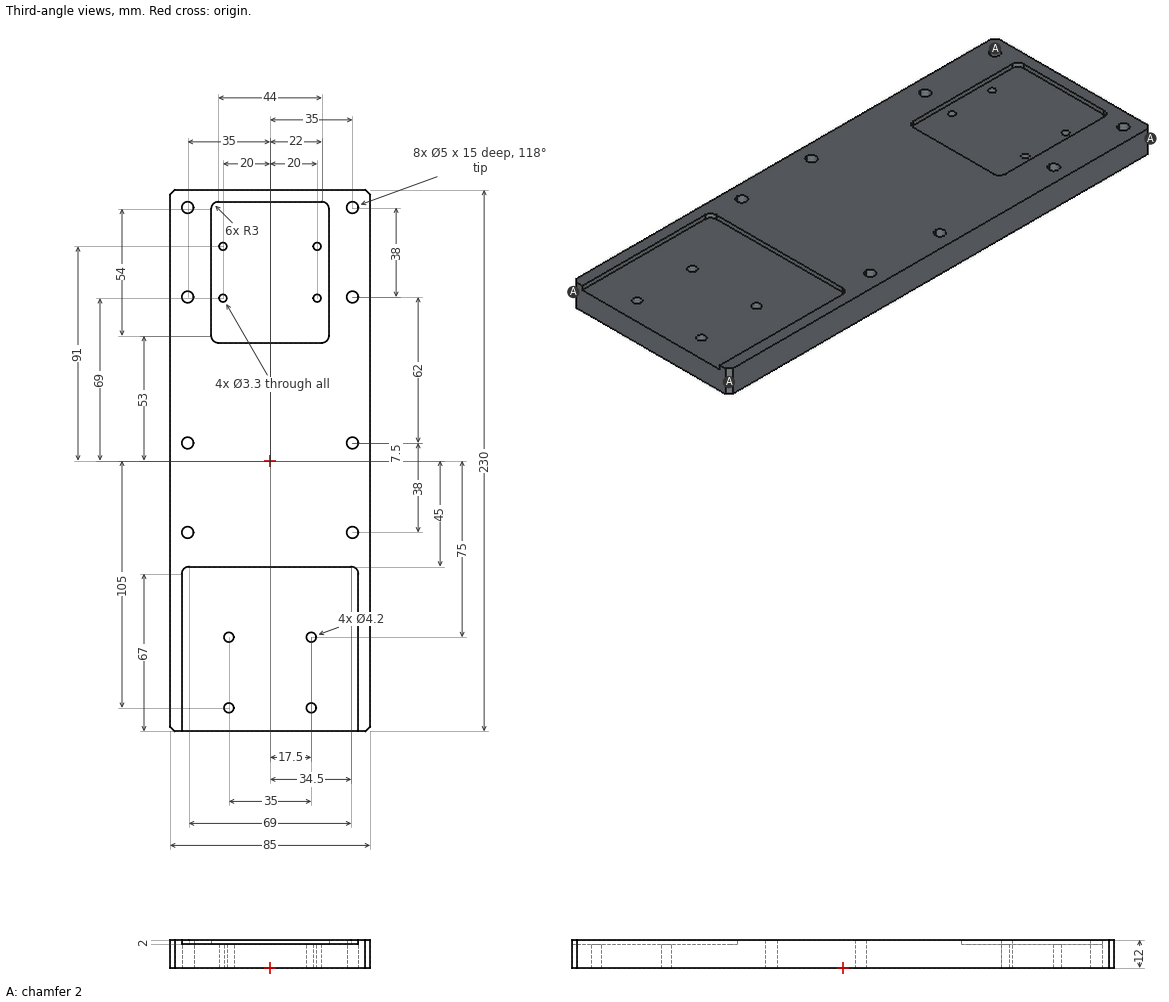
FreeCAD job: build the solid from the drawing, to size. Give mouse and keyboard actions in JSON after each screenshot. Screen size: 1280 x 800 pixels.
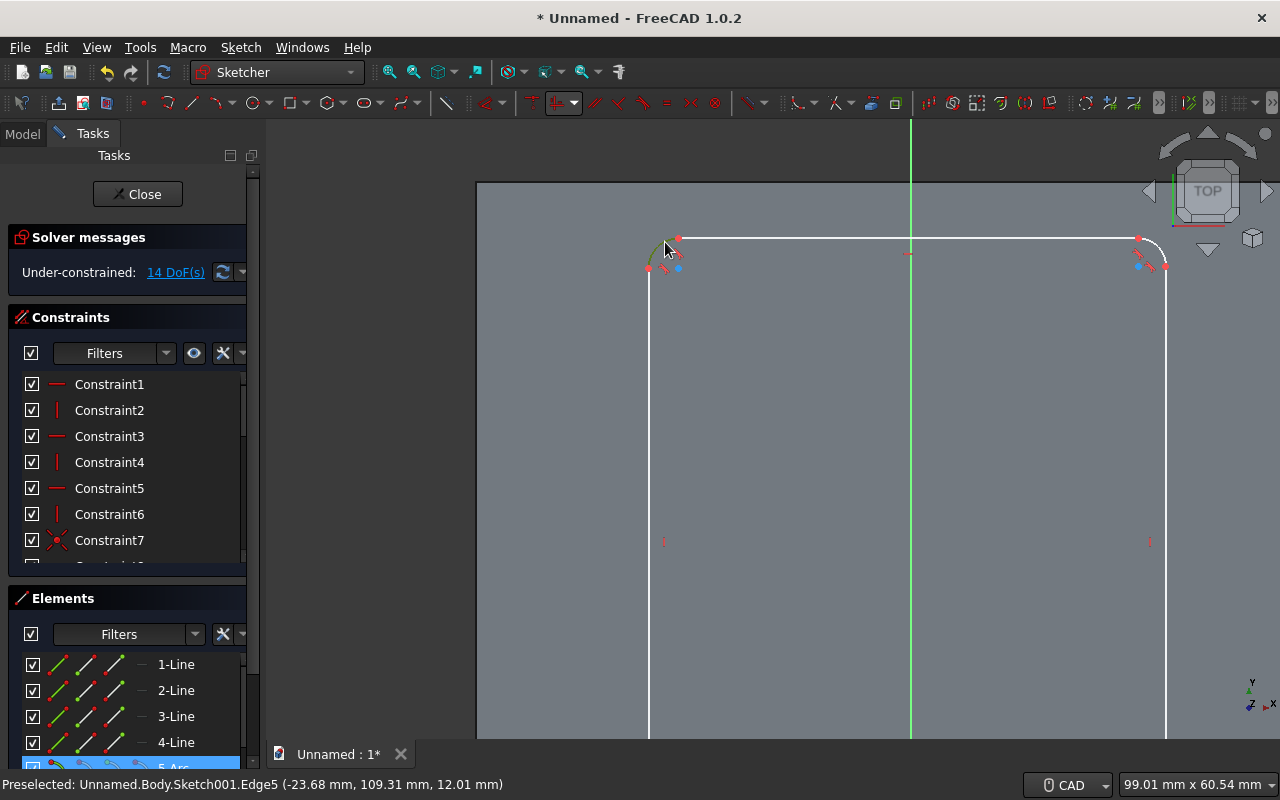
{"action": "scroll", "coordinate": [664, 240], "scroll_direction": "down", "scroll_amount": 9}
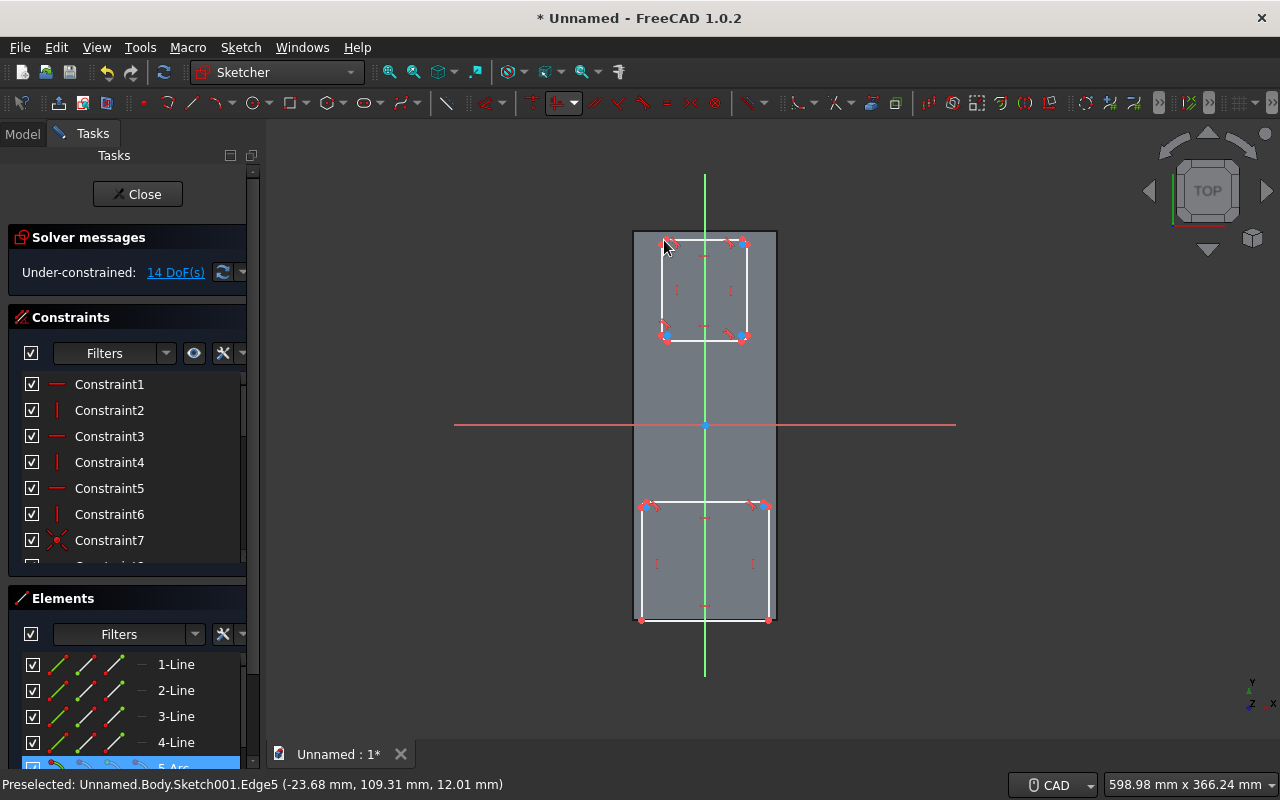
{"action": "scroll", "coordinate": [662, 338], "scroll_direction": "up", "scroll_amount": 8}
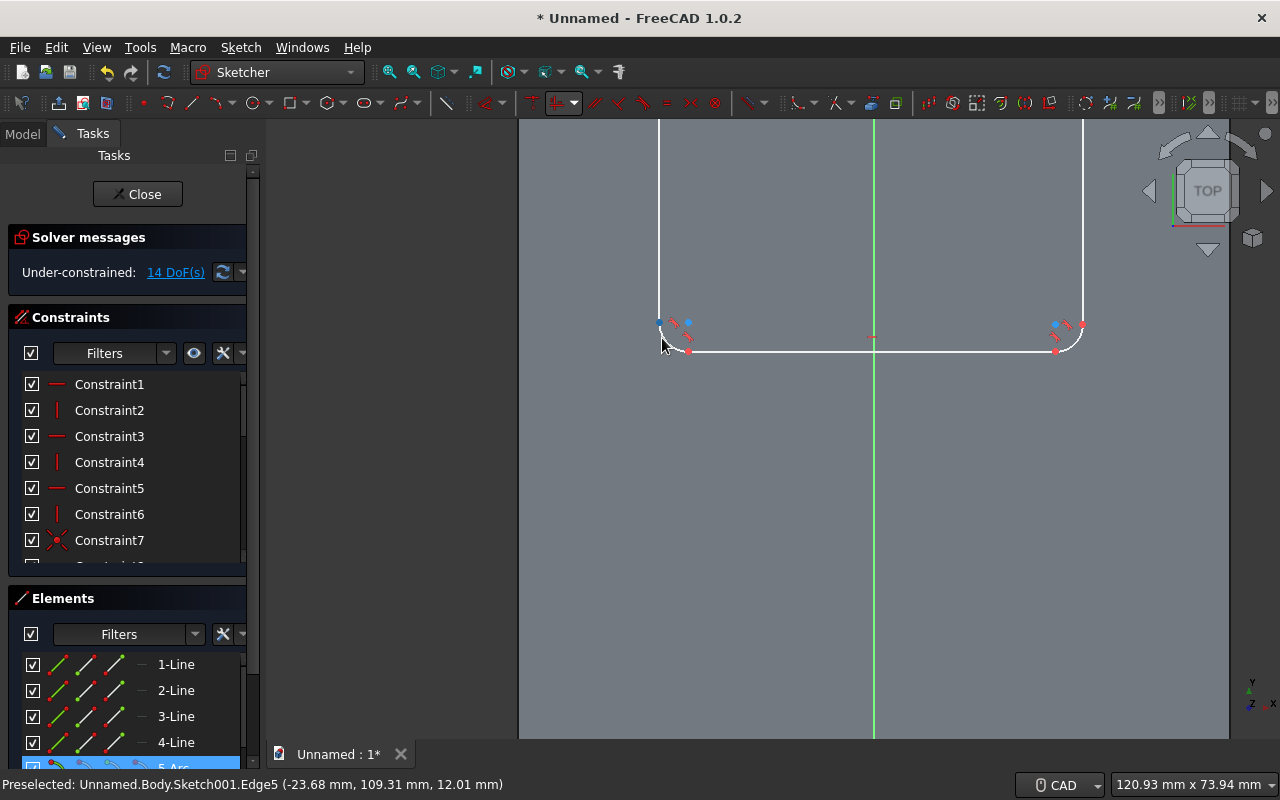
{"action": "left_click", "coordinate": [663, 336]}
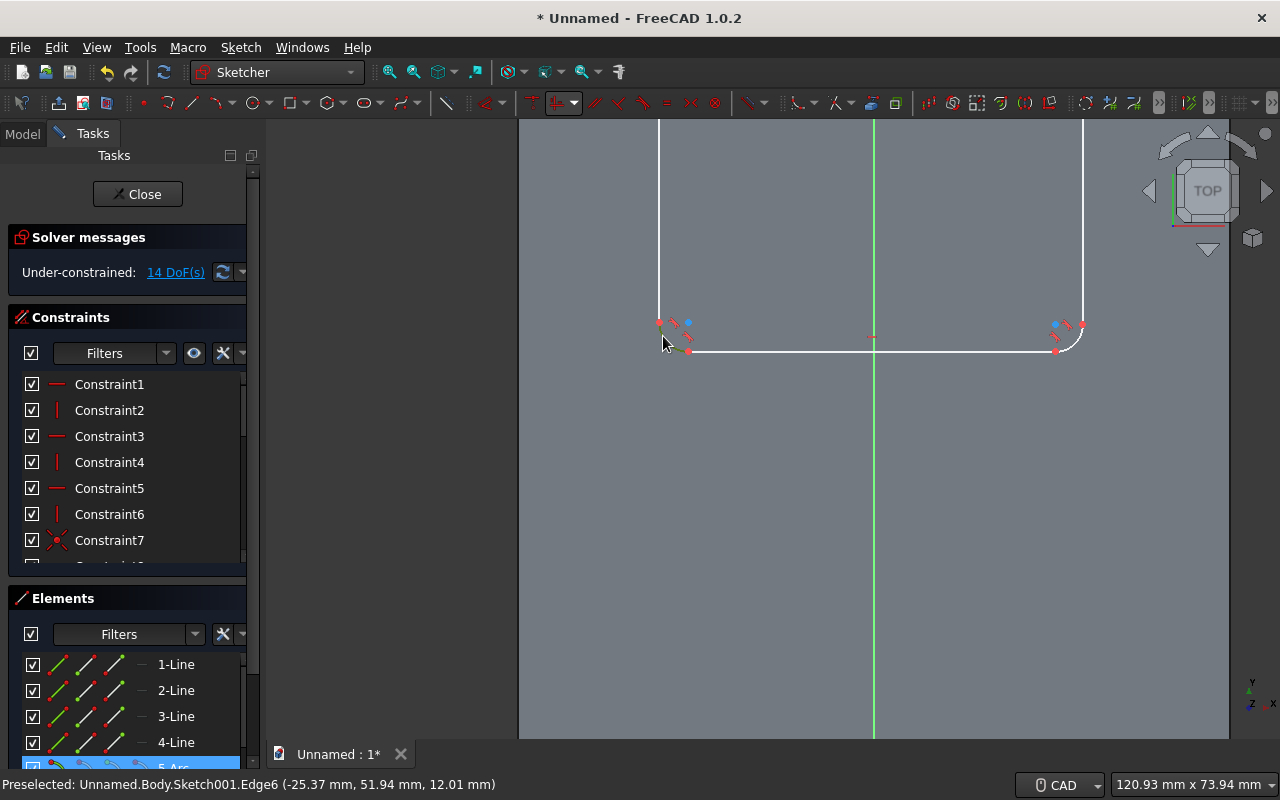
{"action": "left_click", "coordinate": [1068, 349]}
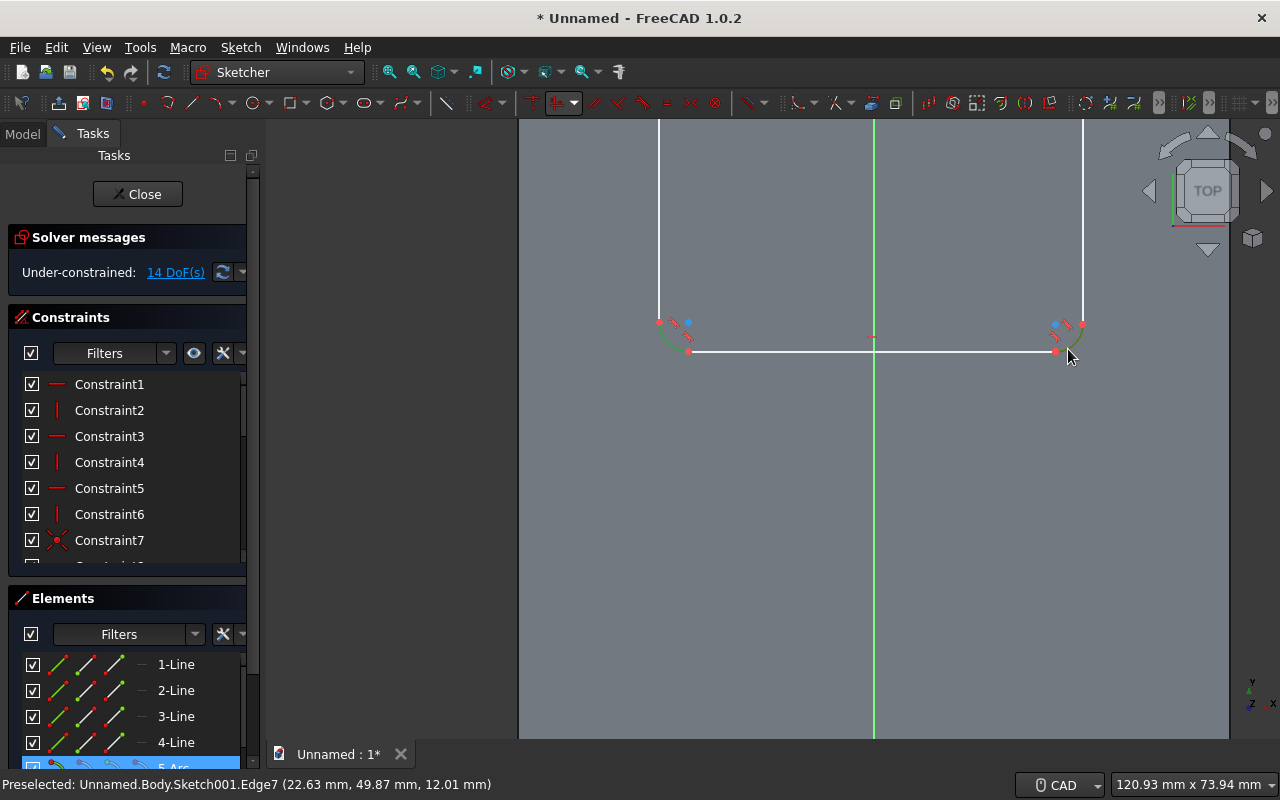
{"action": "scroll", "coordinate": [662, 338], "scroll_direction": "down", "scroll_amount": 8}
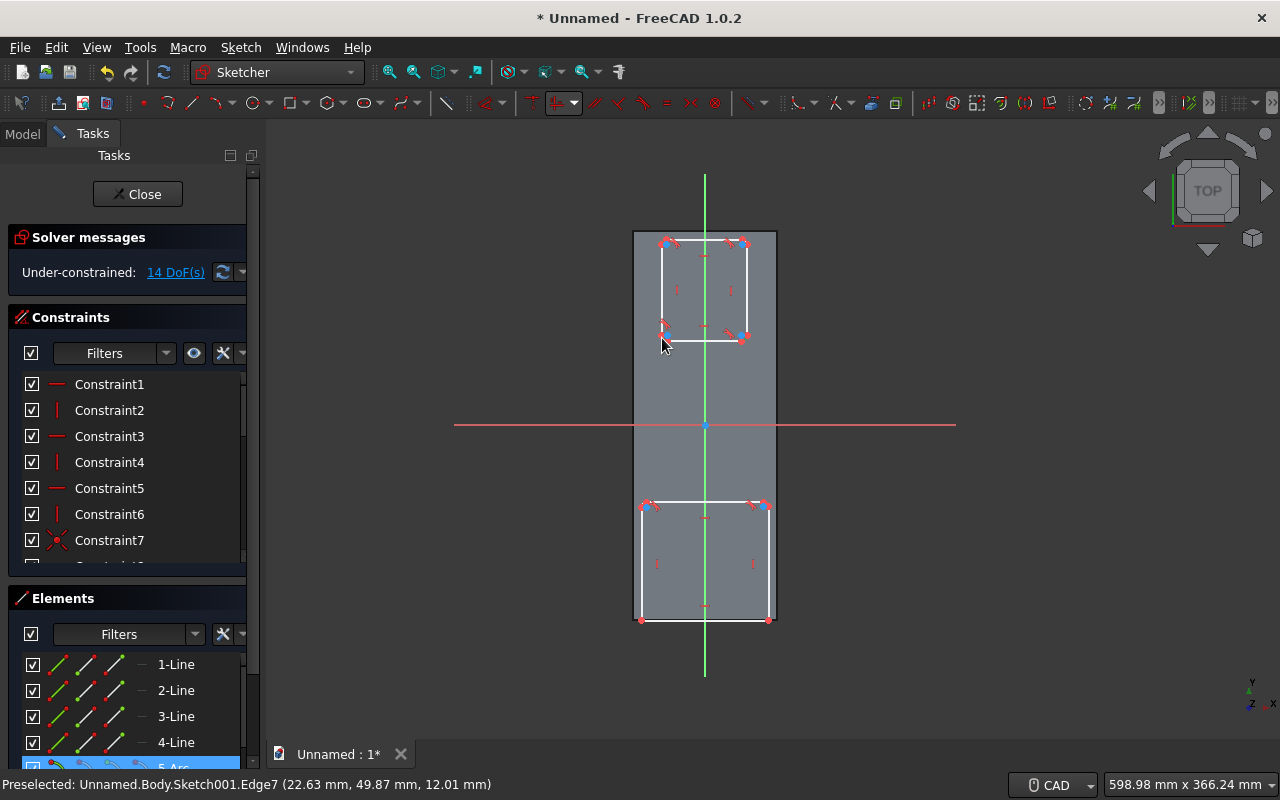
{"action": "scroll", "coordinate": [747, 242], "scroll_direction": "up", "scroll_amount": 10}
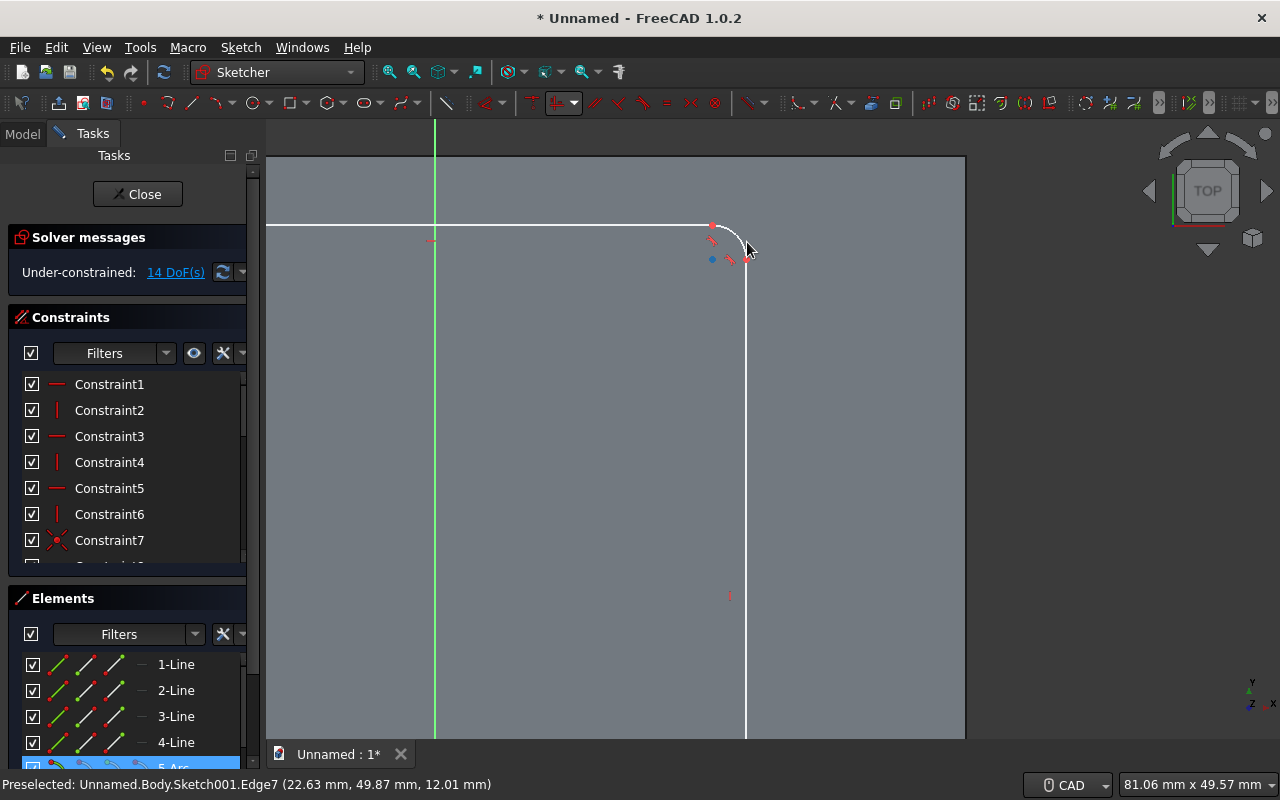
{"action": "left_click", "coordinate": [743, 244]}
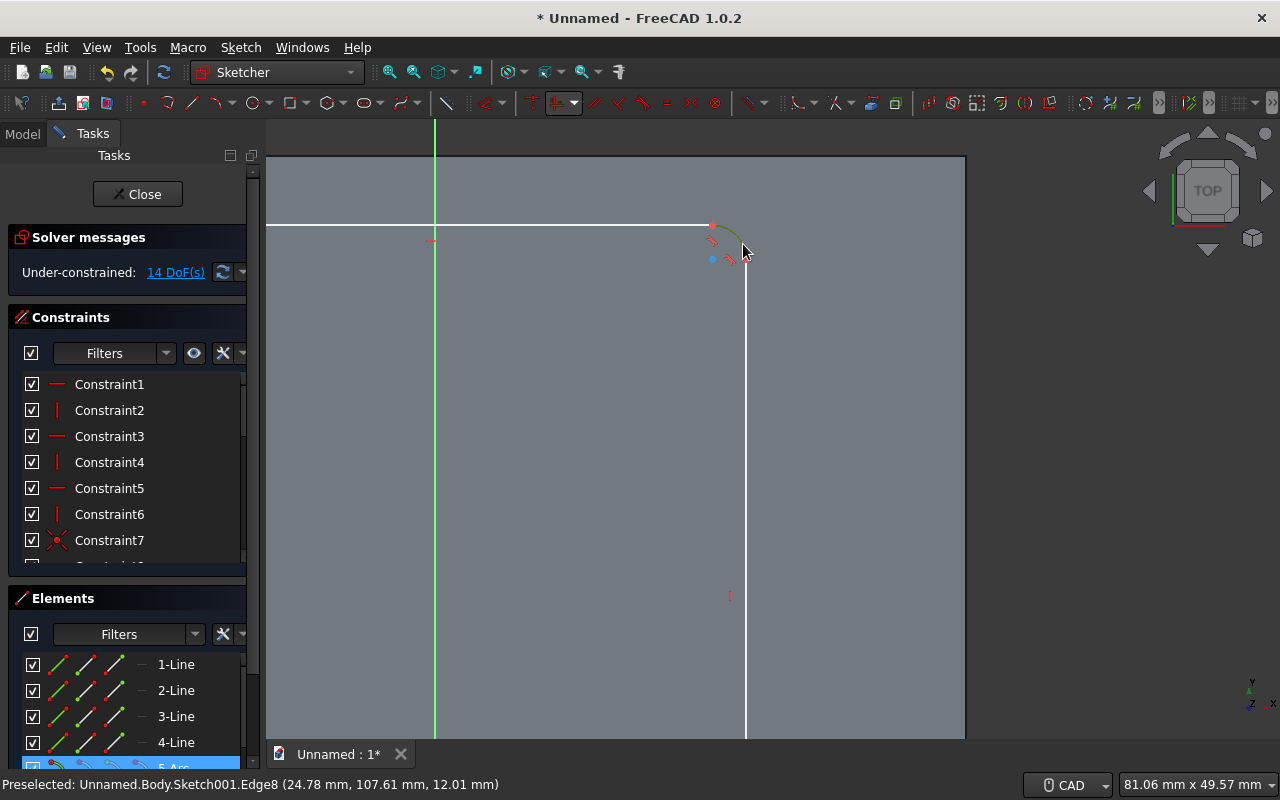
{"action": "scroll", "coordinate": [747, 242], "scroll_direction": "down", "scroll_amount": 10}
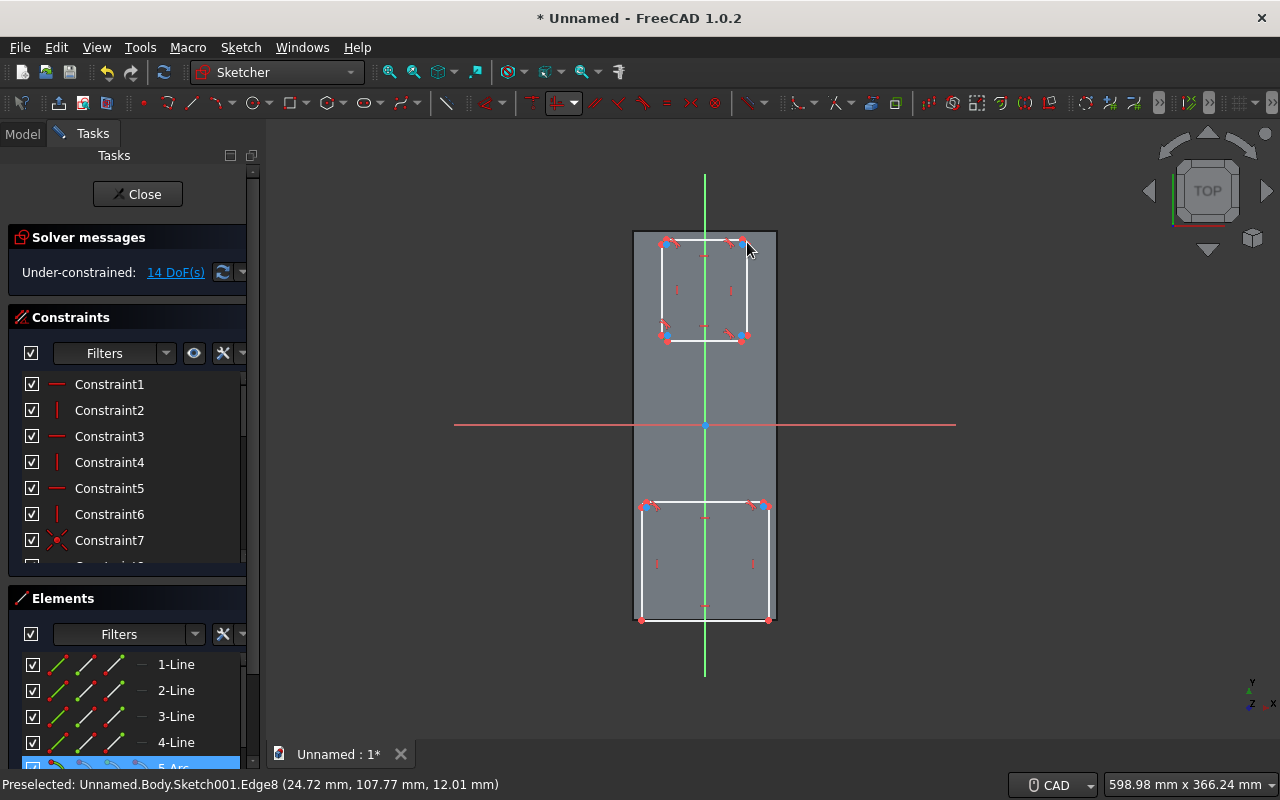
{"action": "scroll", "coordinate": [645, 503], "scroll_direction": "up", "scroll_amount": 9}